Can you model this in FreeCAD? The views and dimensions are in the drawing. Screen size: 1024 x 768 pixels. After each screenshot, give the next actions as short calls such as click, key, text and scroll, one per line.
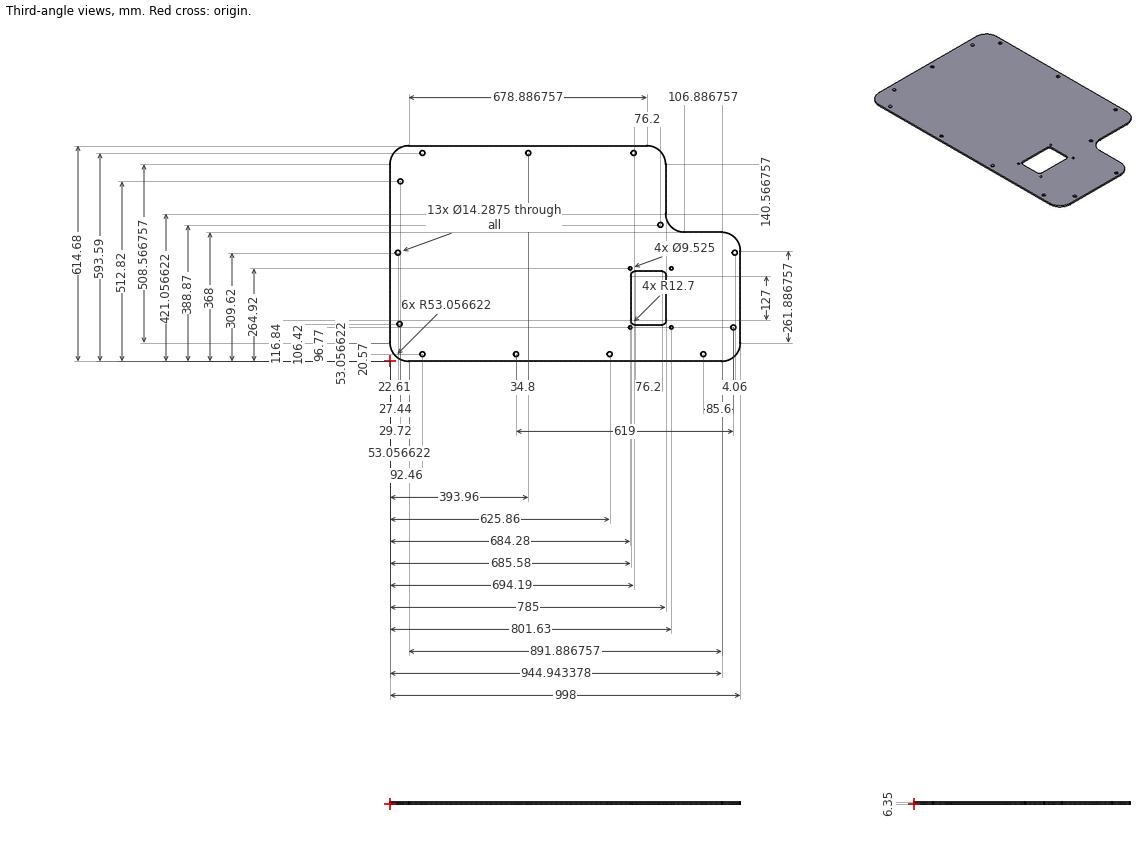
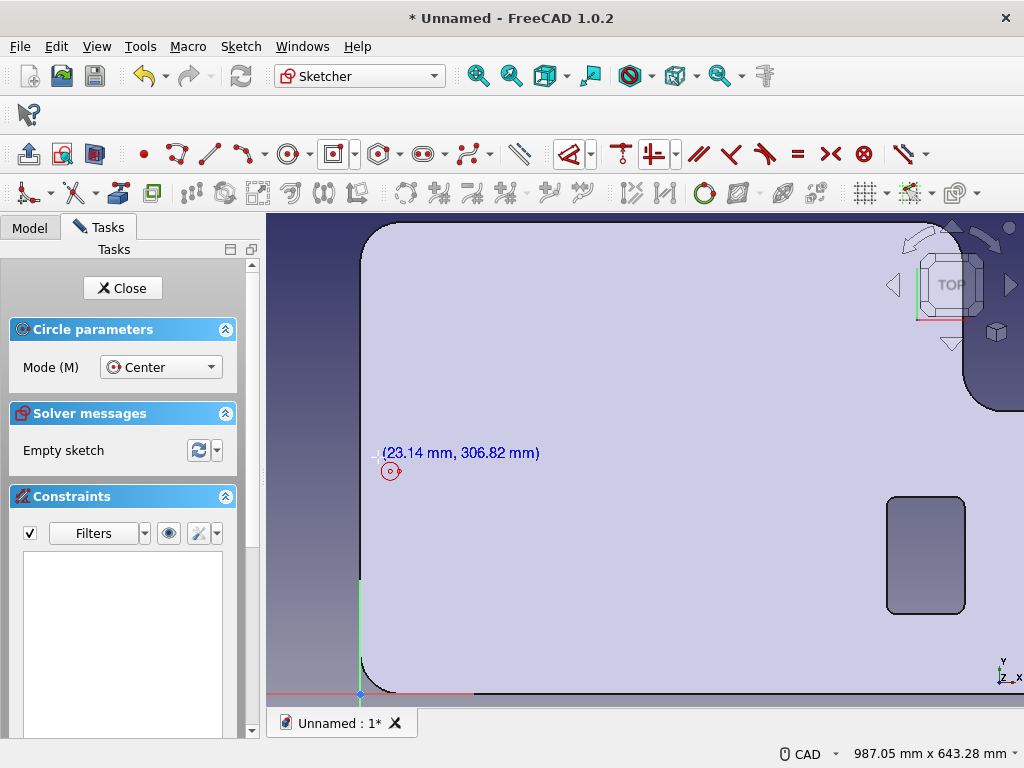
click(377, 456)
move(381, 452)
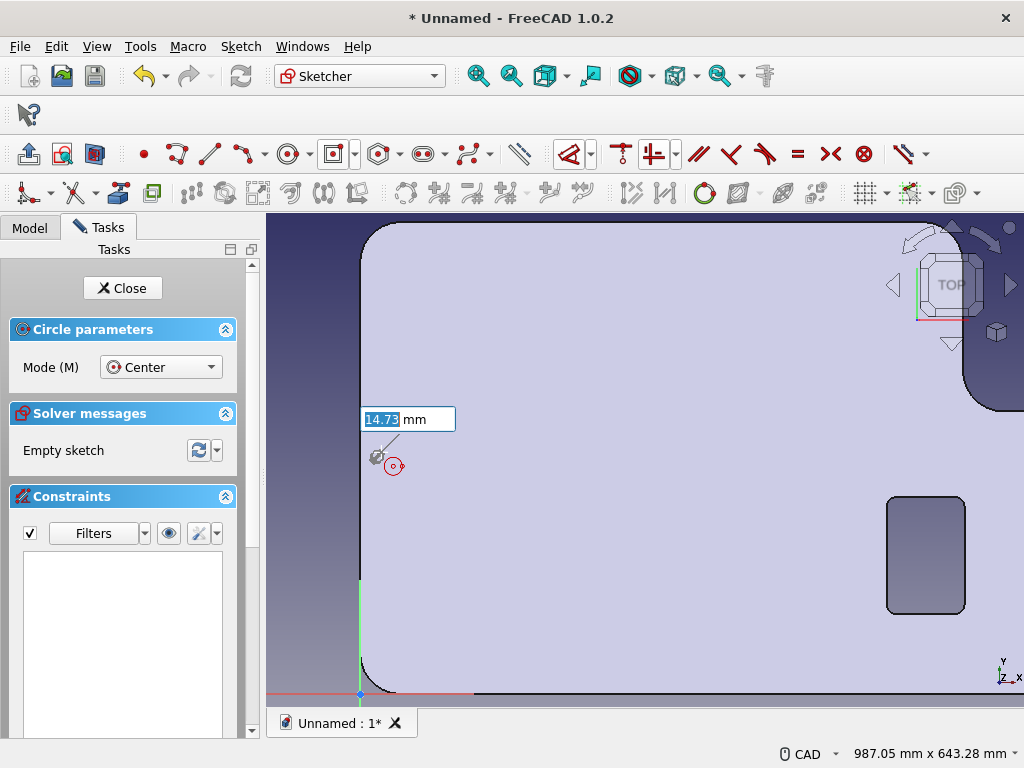
text(14.2875)
key(Return)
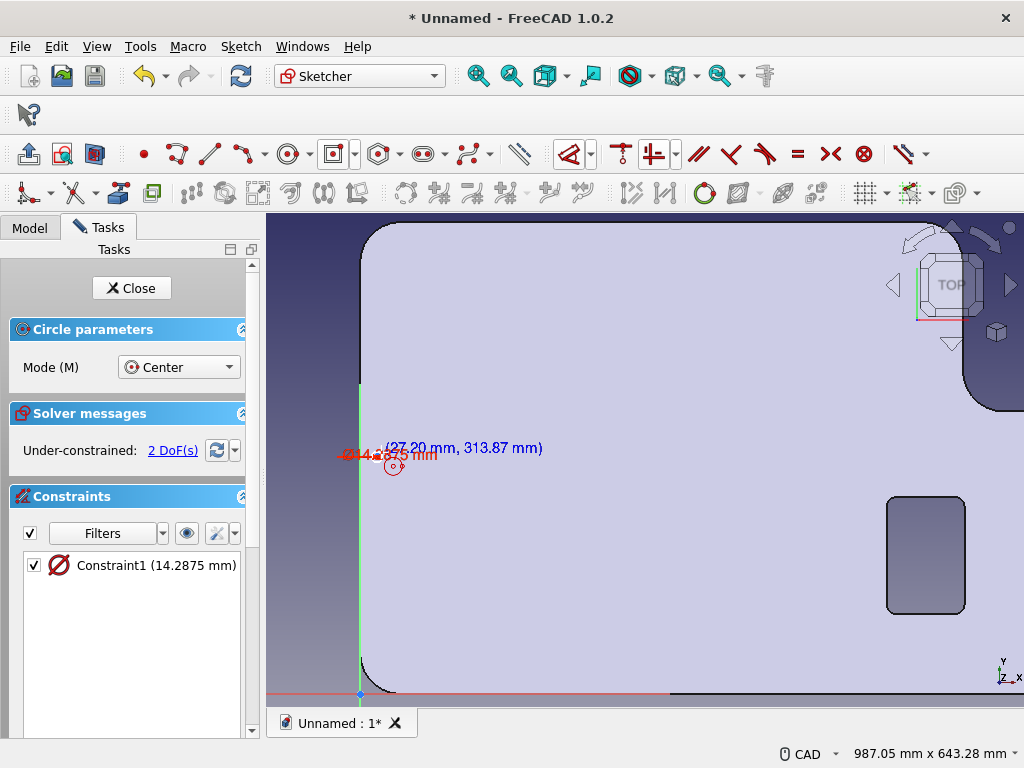
scroll(383, 300, up, 8)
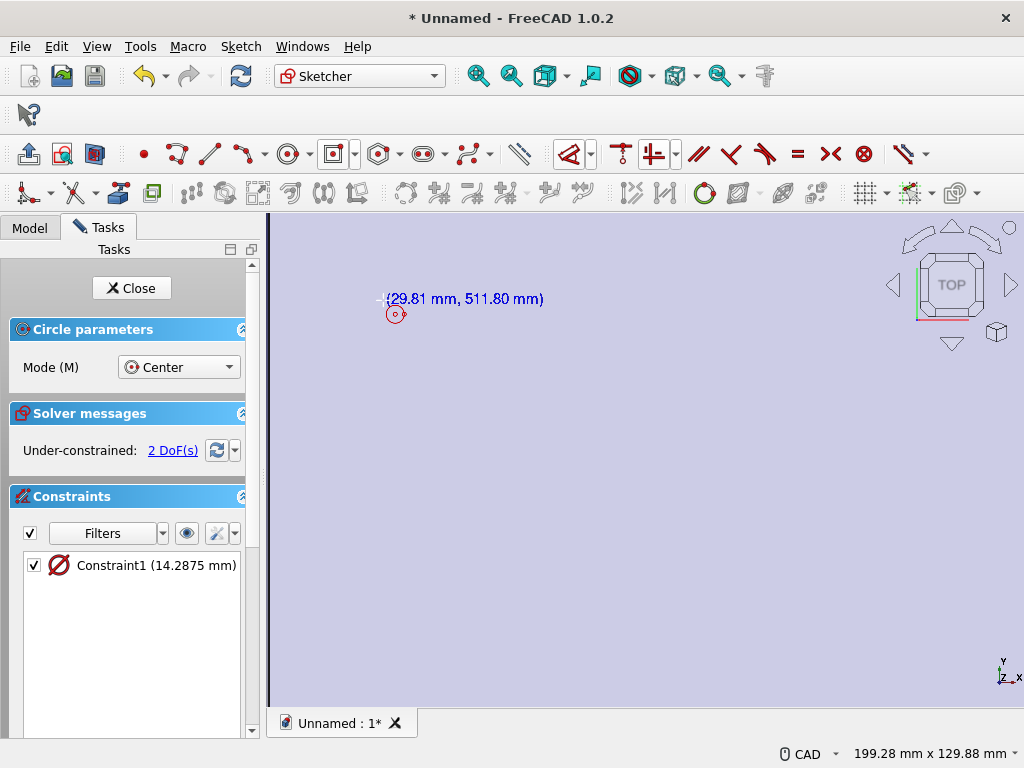
scroll(380, 379, down, 11)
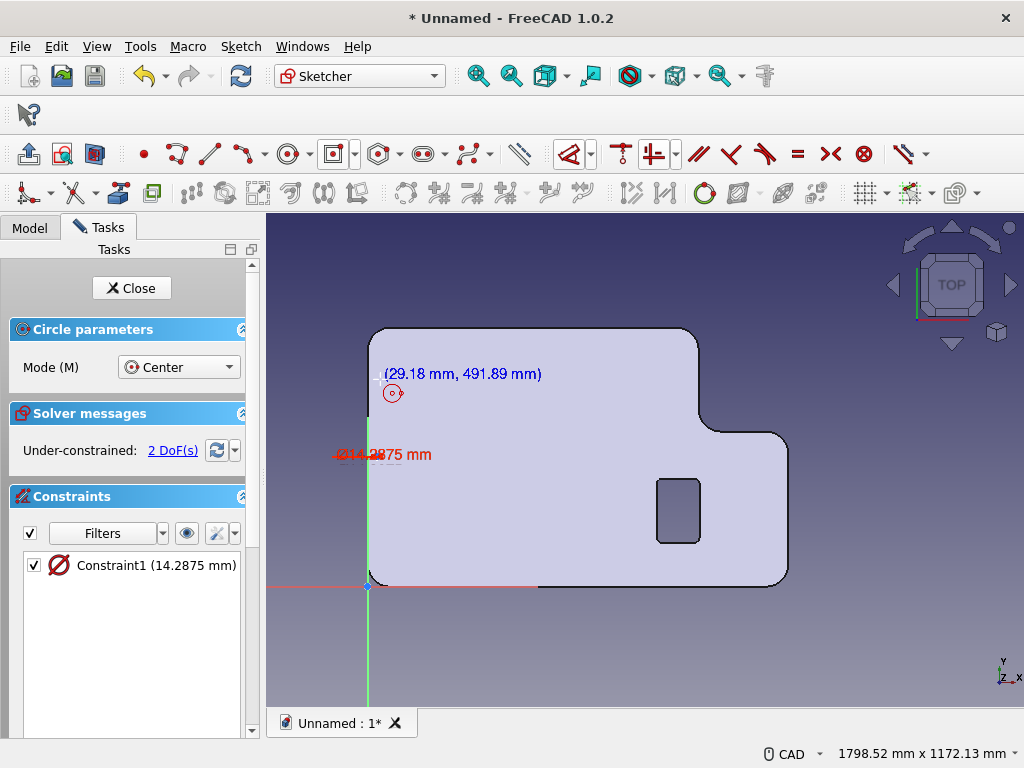
scroll(380, 371, up, 2)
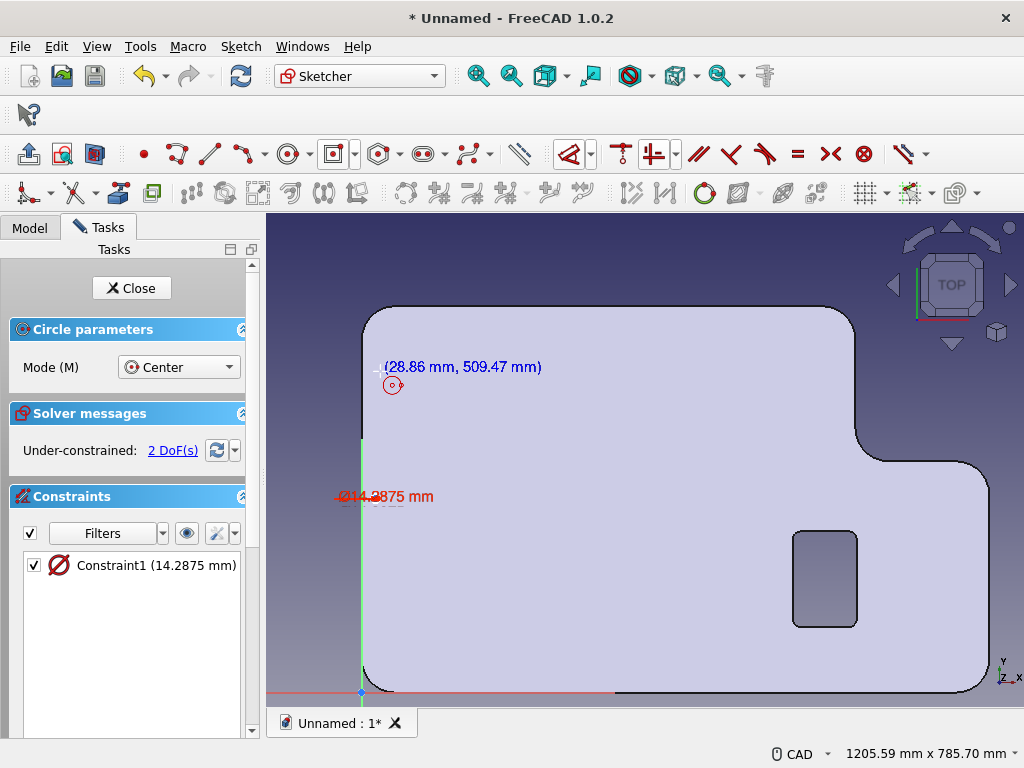
click(380, 370)
move(384, 367)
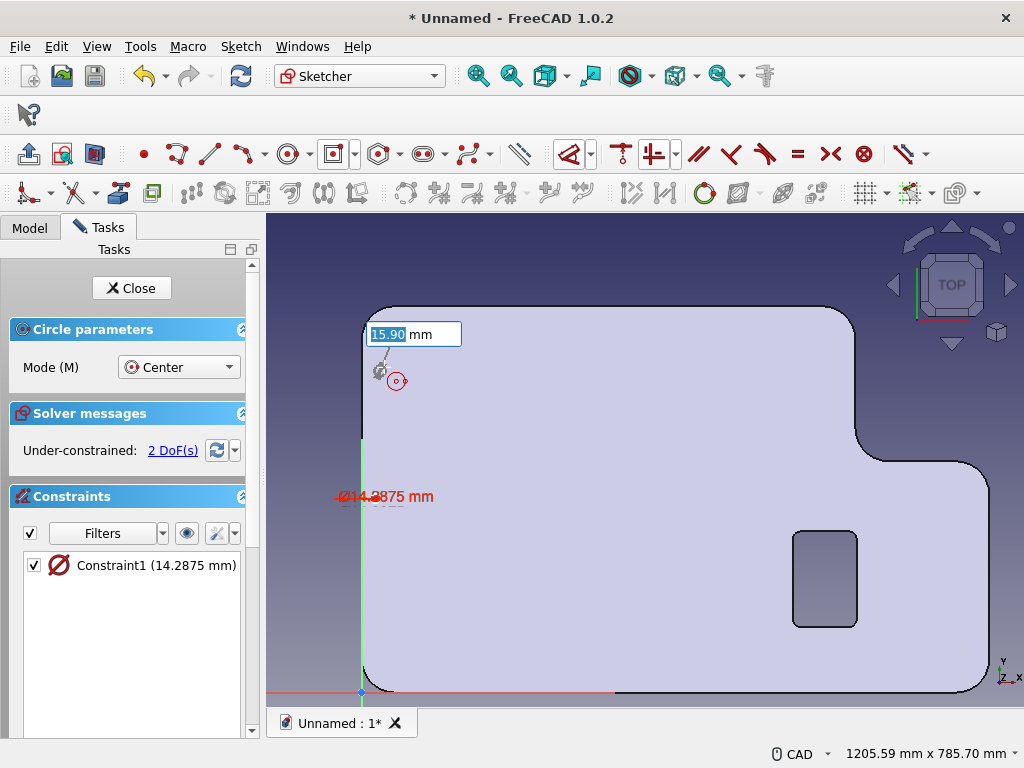
text(14.2875)
key(Return)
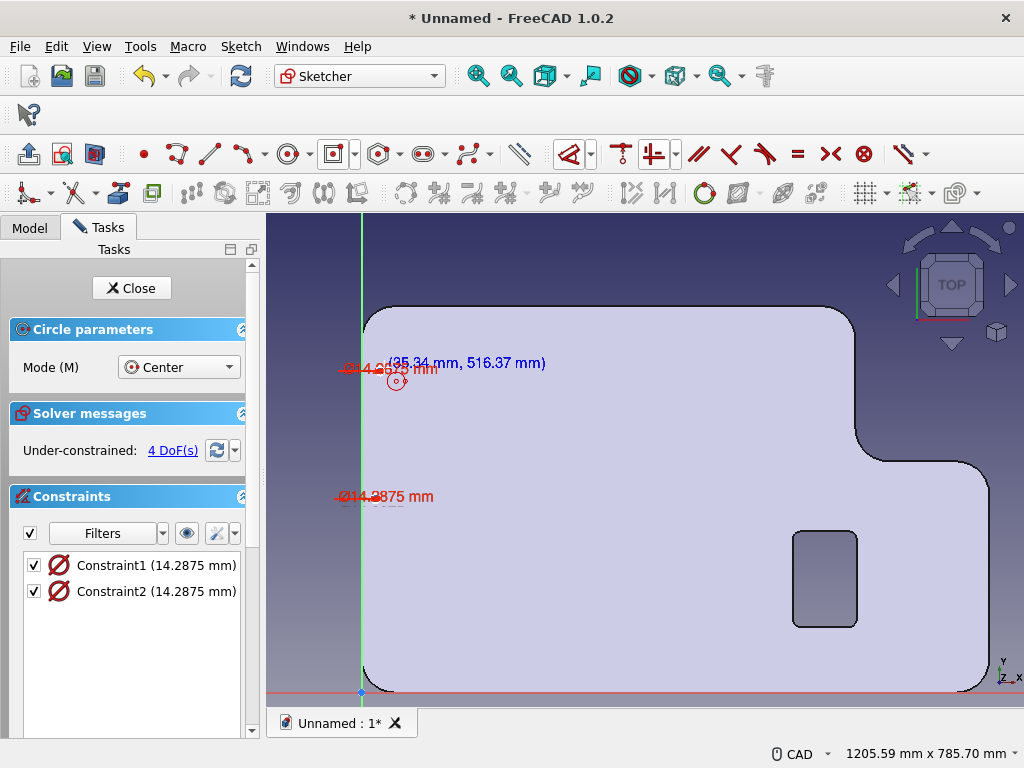
scroll(379, 626, up, 9)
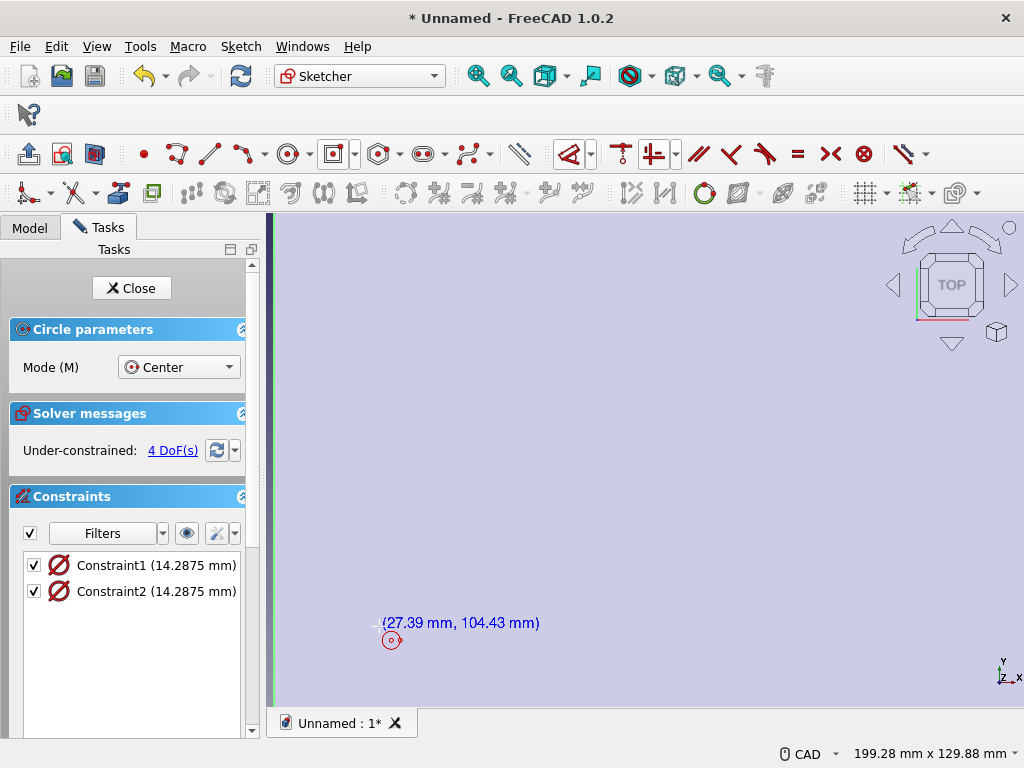
scroll(380, 532, down, 11)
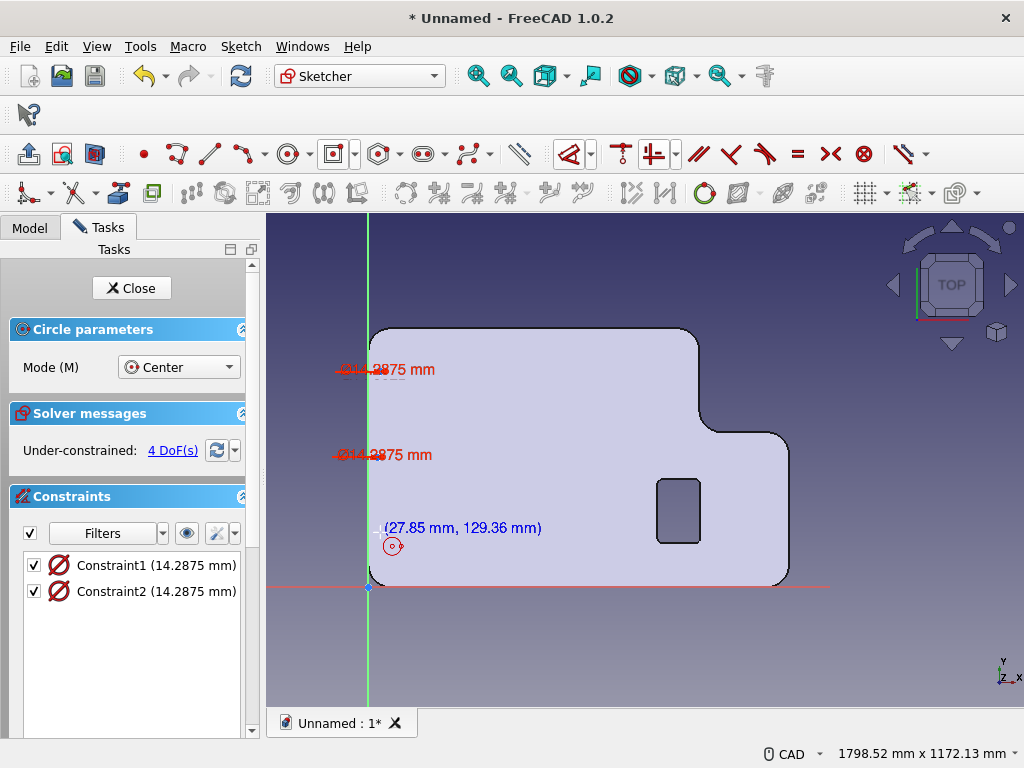
scroll(380, 542, up, 2)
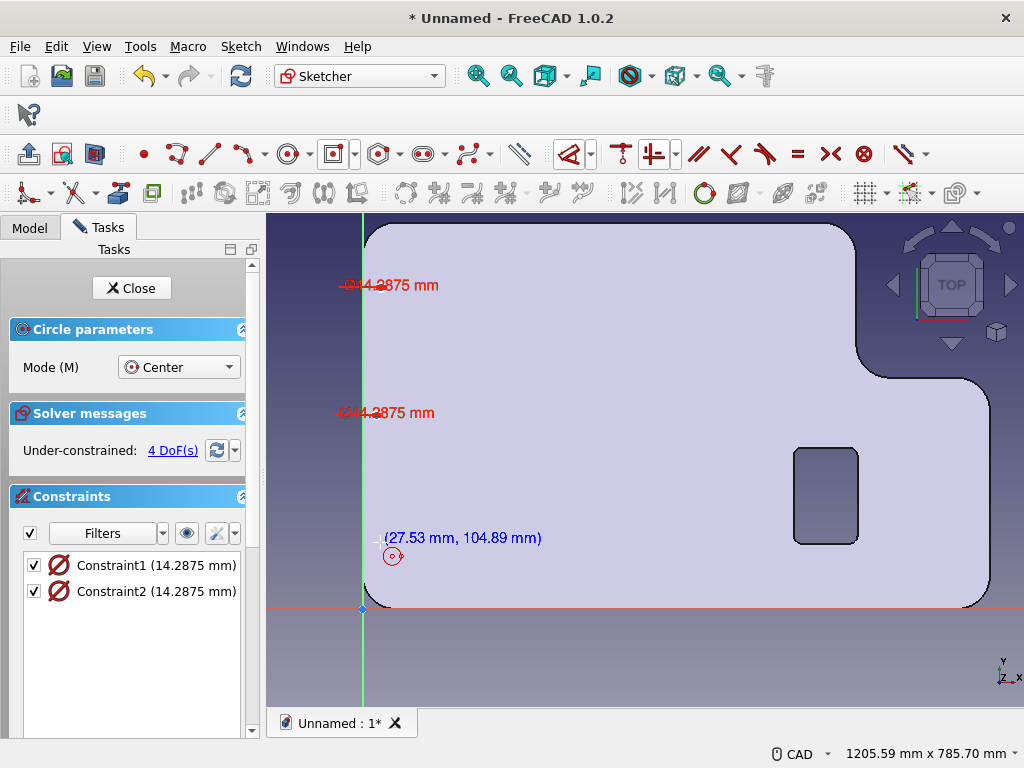
click(380, 542)
move(383, 539)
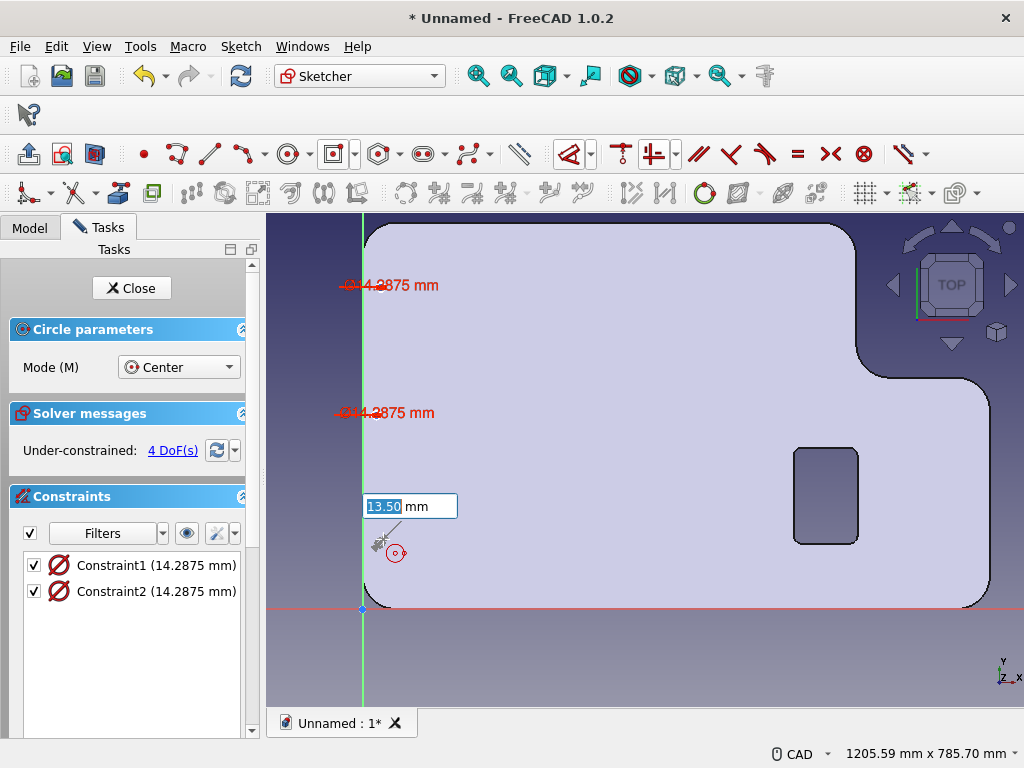
text(14.2875)
key(Return)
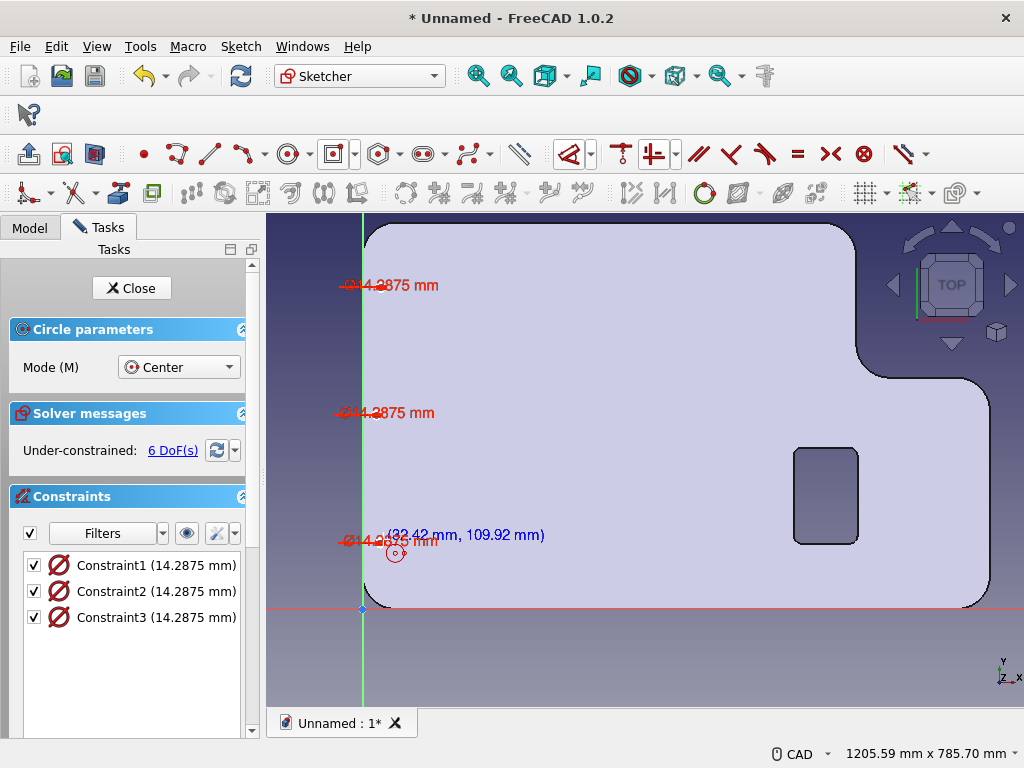
scroll(421, 596, up, 9)